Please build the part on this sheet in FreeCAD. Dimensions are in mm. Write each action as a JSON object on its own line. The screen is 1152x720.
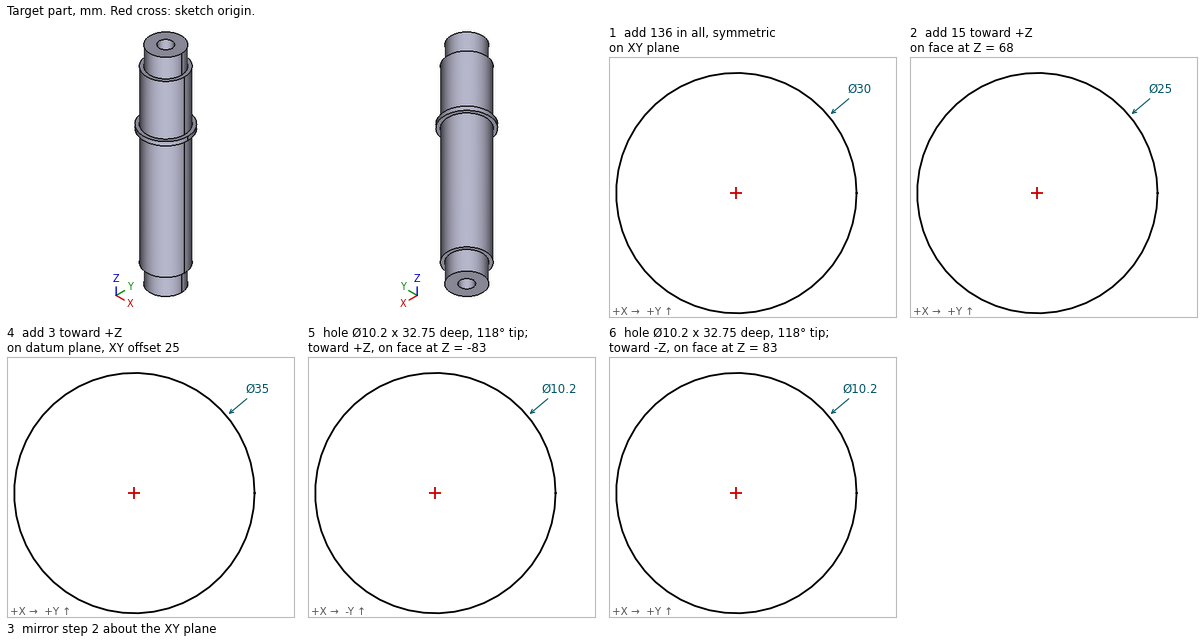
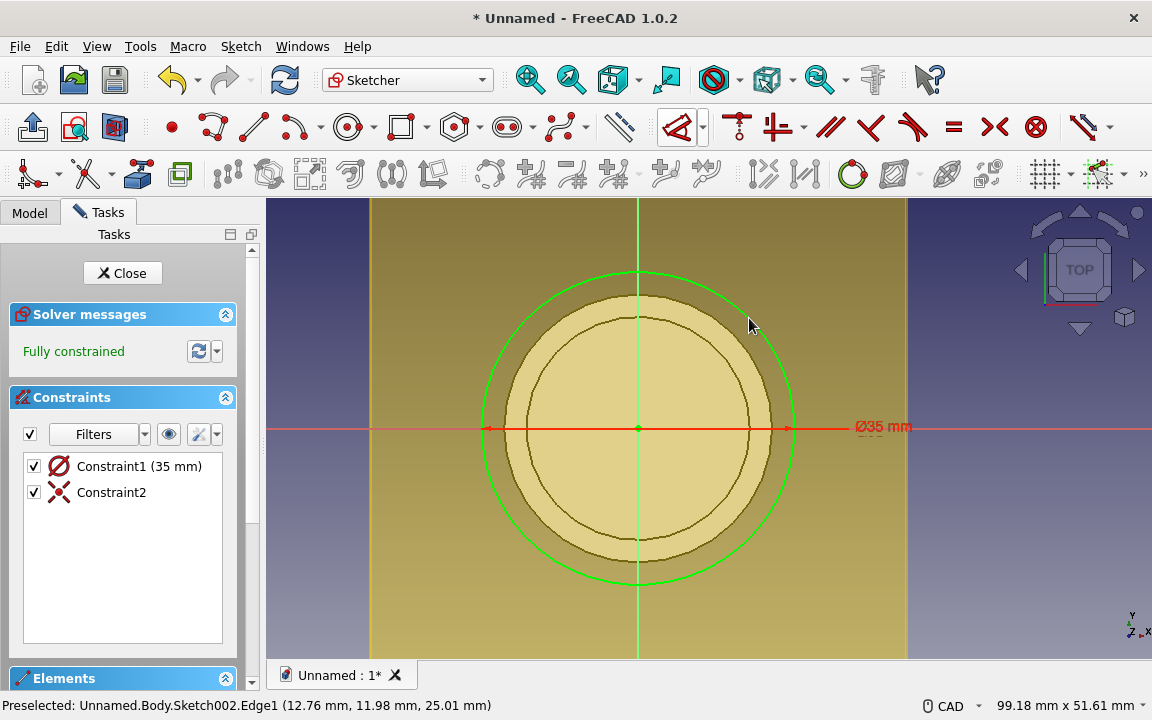
{"action": "left_click", "coordinate": [123, 273]}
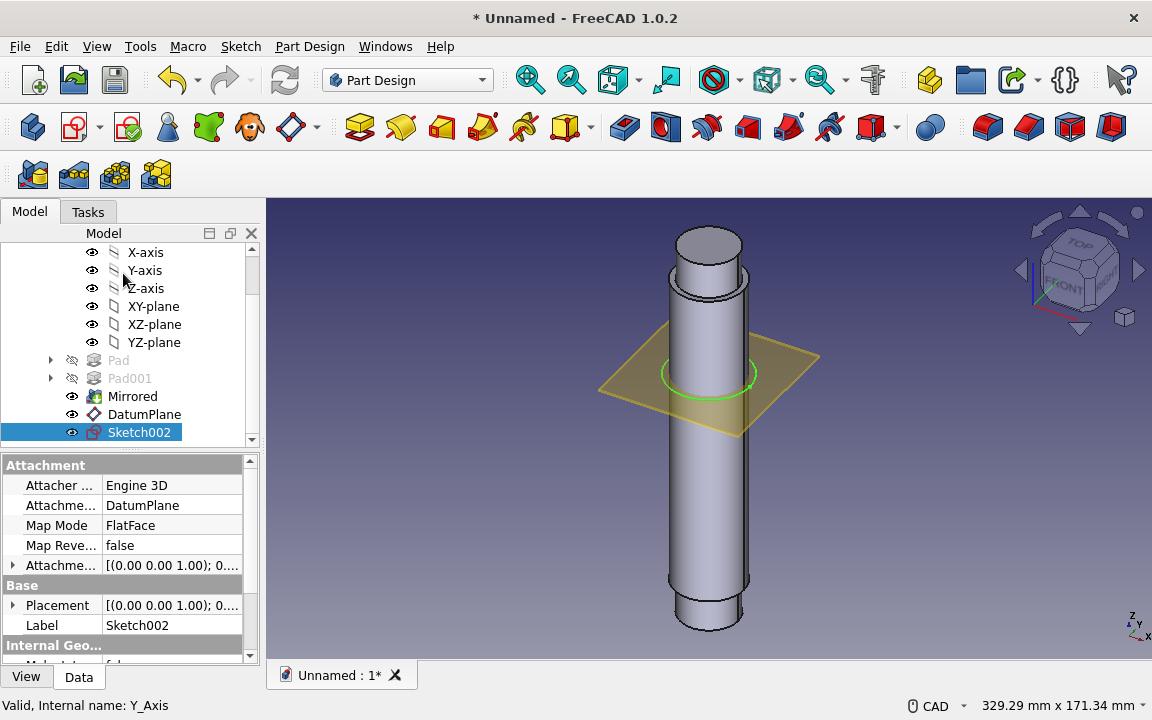
{"action": "left_click", "coordinate": [360, 128]}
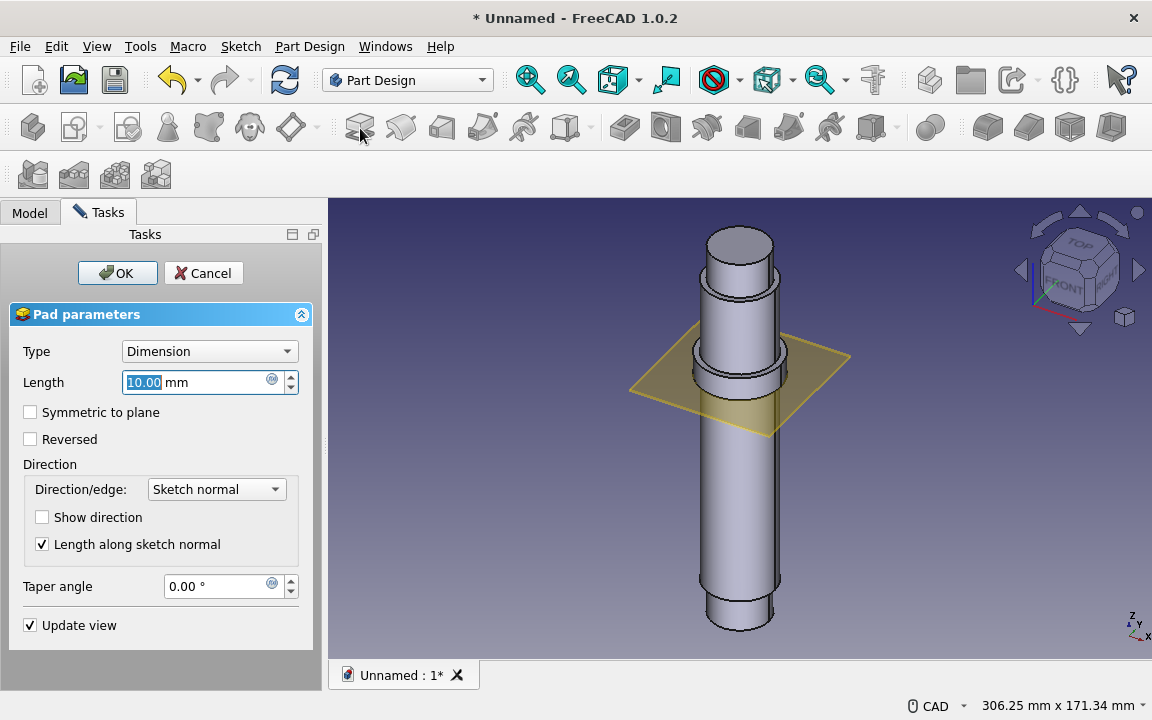
{"action": "type", "text": "3"}
{"action": "key", "text": "Tab"}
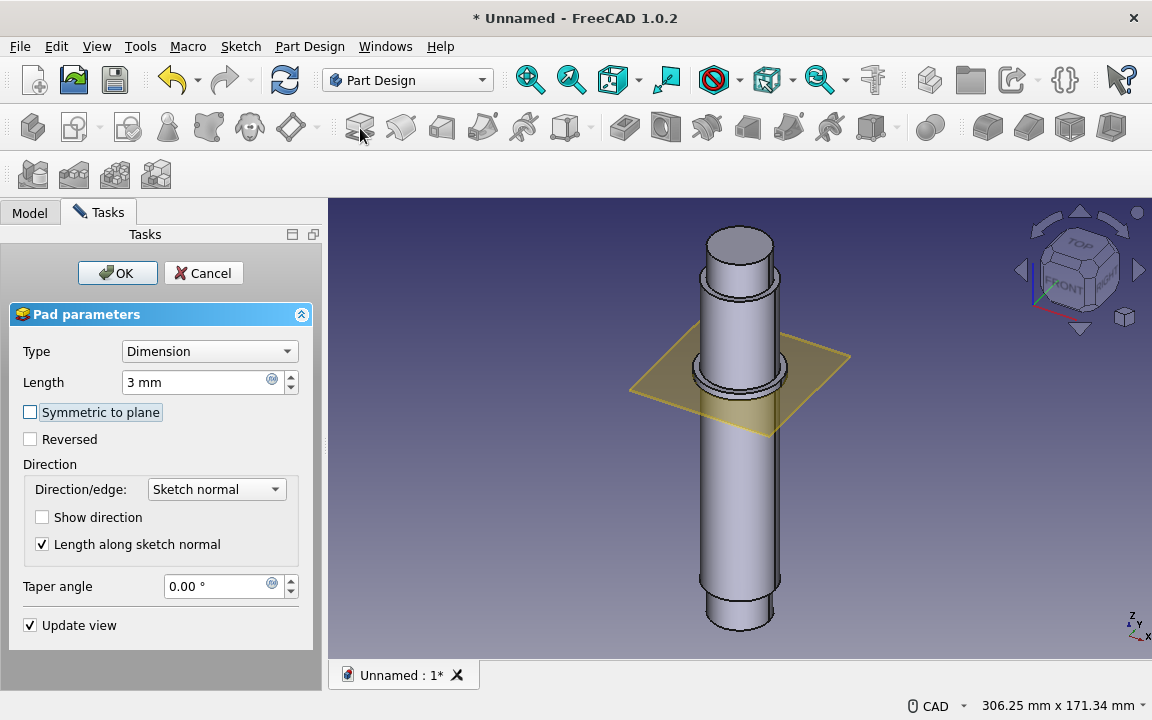
{"action": "left_click", "coordinate": [118, 273]}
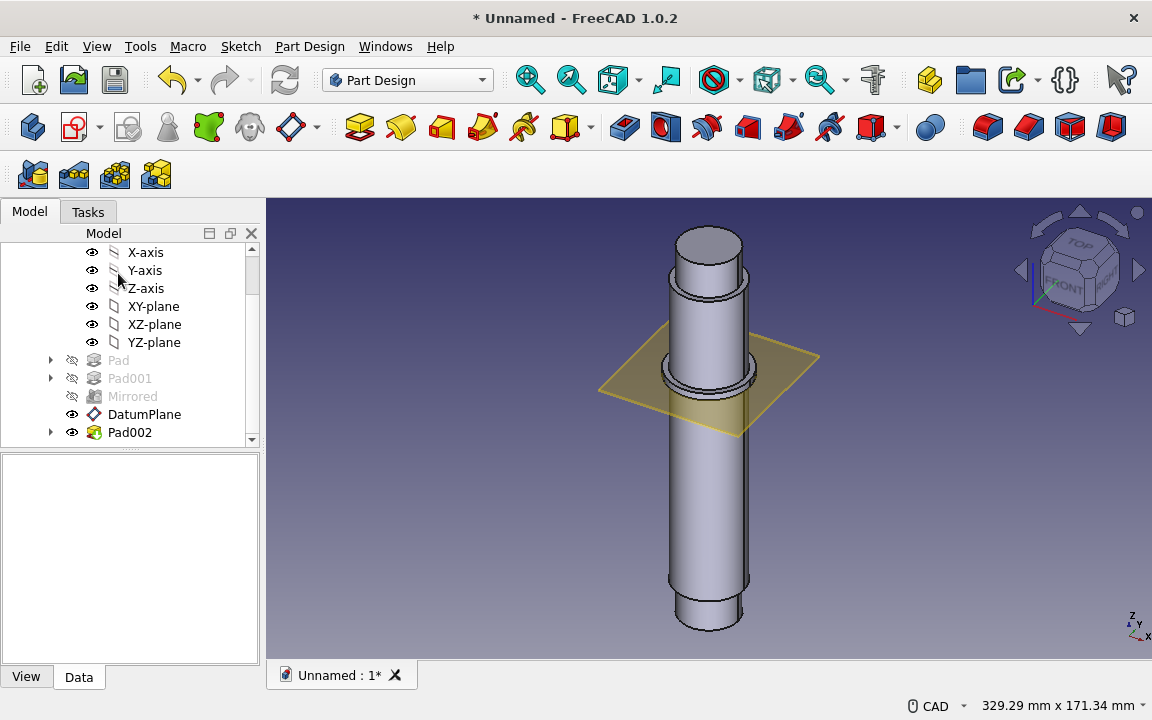
{"action": "left_click", "coordinate": [117, 414]}
{"action": "key", "text": "space"}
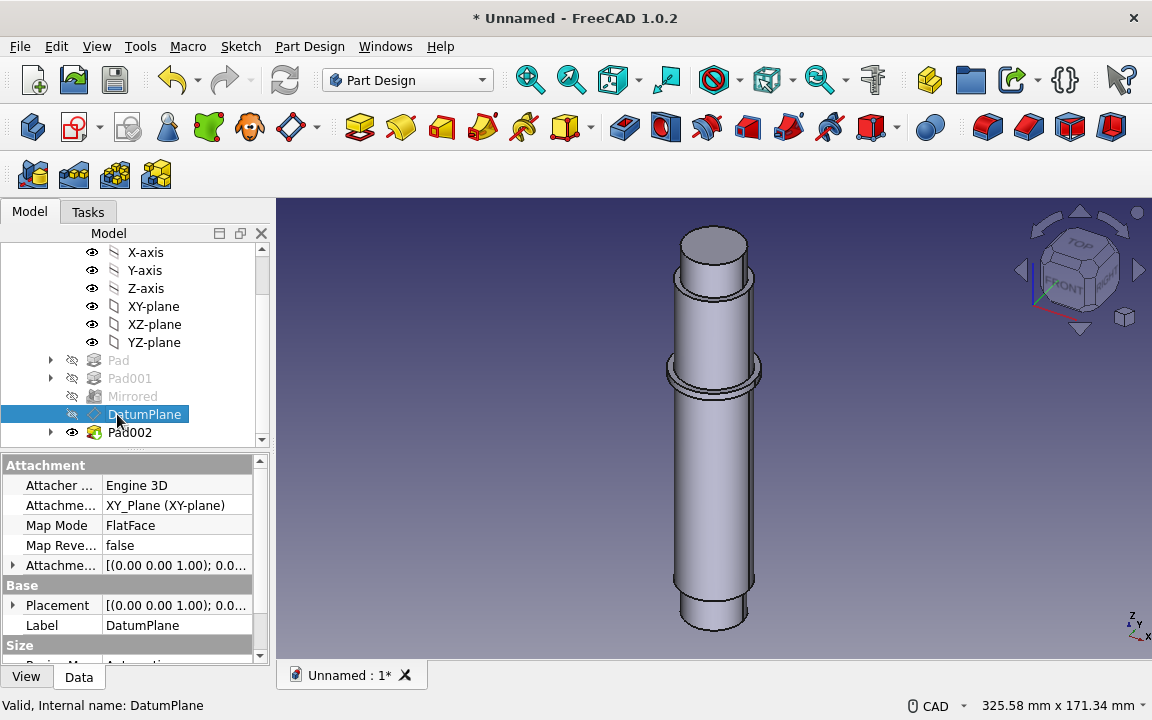
{"action": "key", "text": "5"}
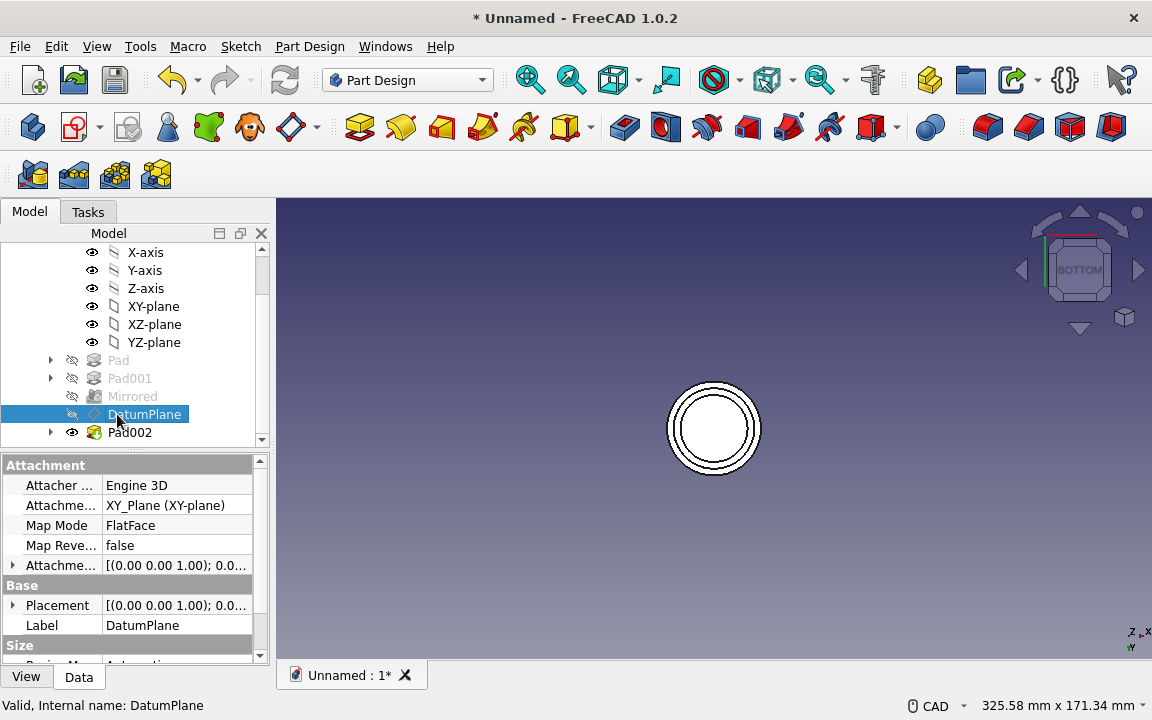
{"action": "left_click", "coordinate": [531, 80]}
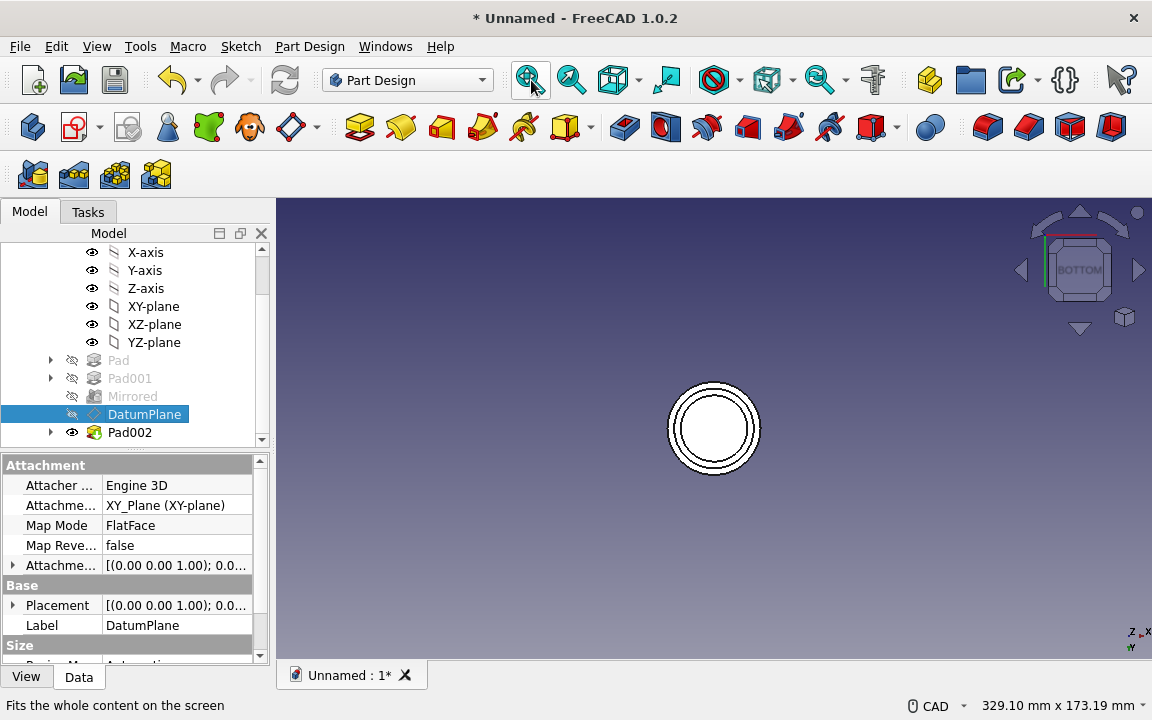
{"action": "left_click", "coordinate": [714, 427]}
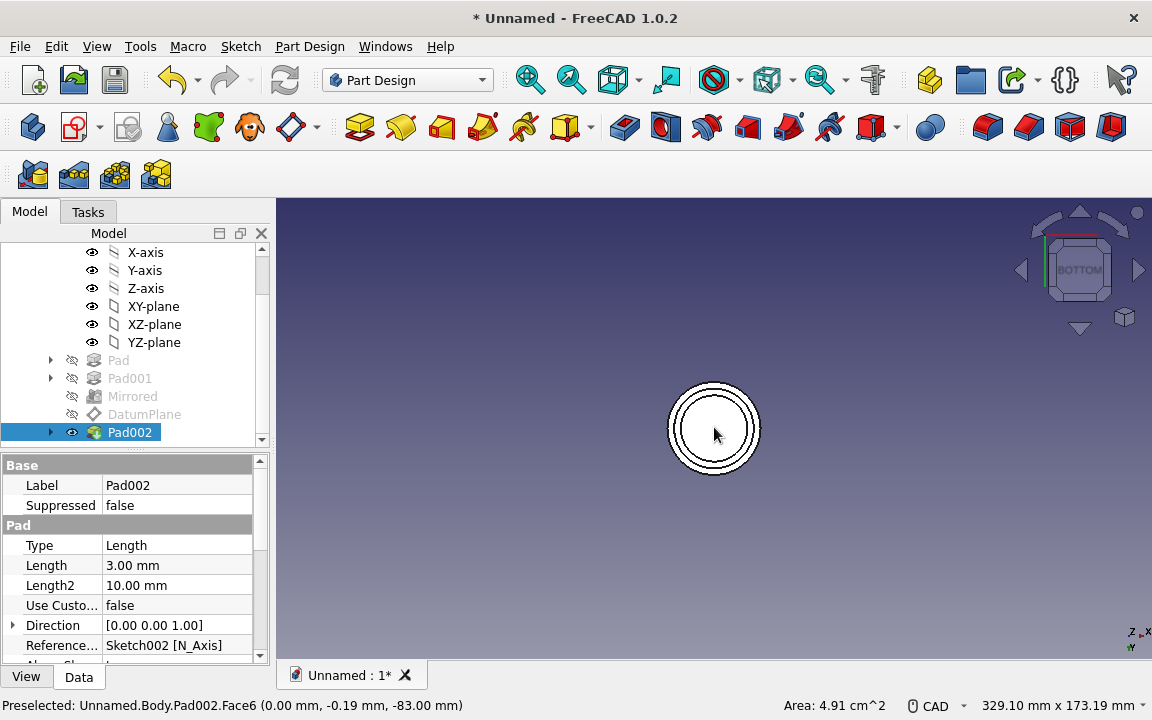
{"action": "left_click", "coordinate": [74, 128]}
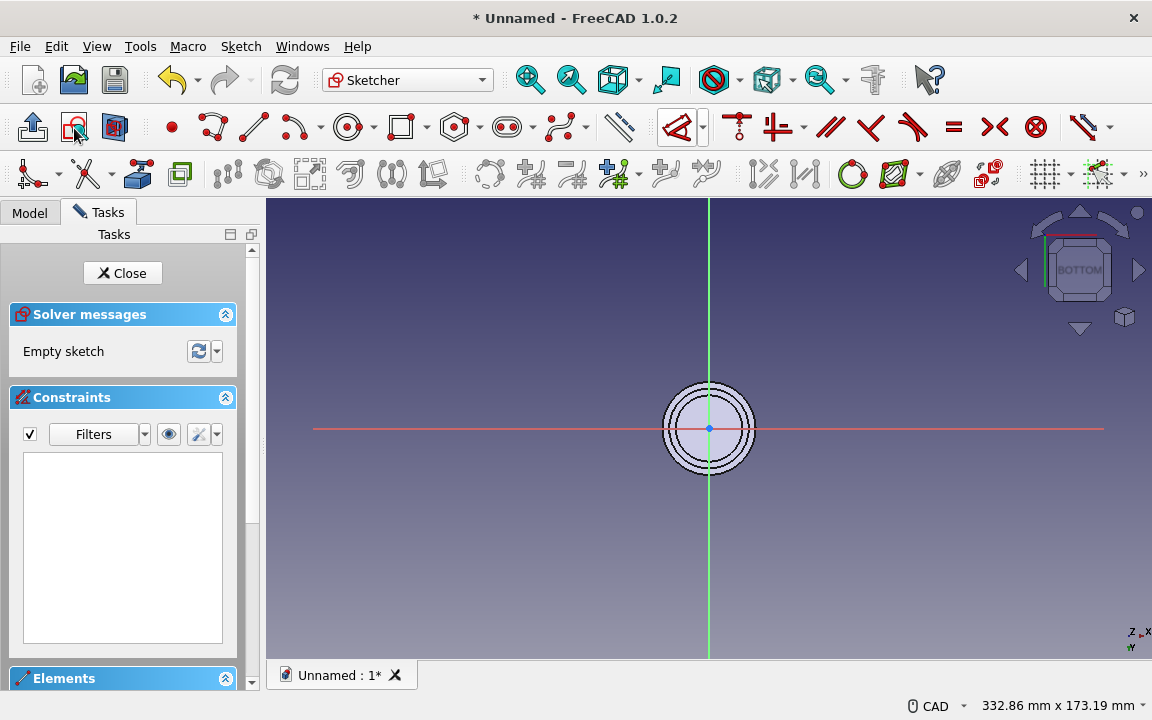
{"action": "scroll", "coordinate": [716, 428], "scroll_direction": "up", "scroll_amount": 12}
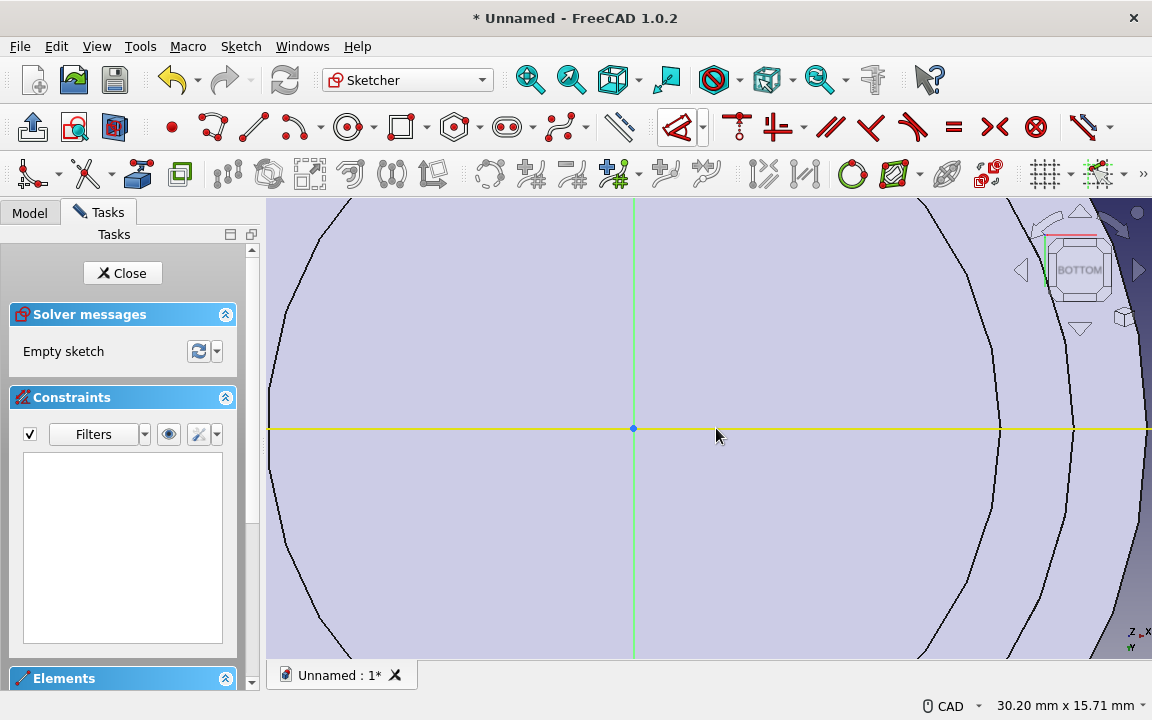
{"action": "left_click", "coordinate": [348, 128]}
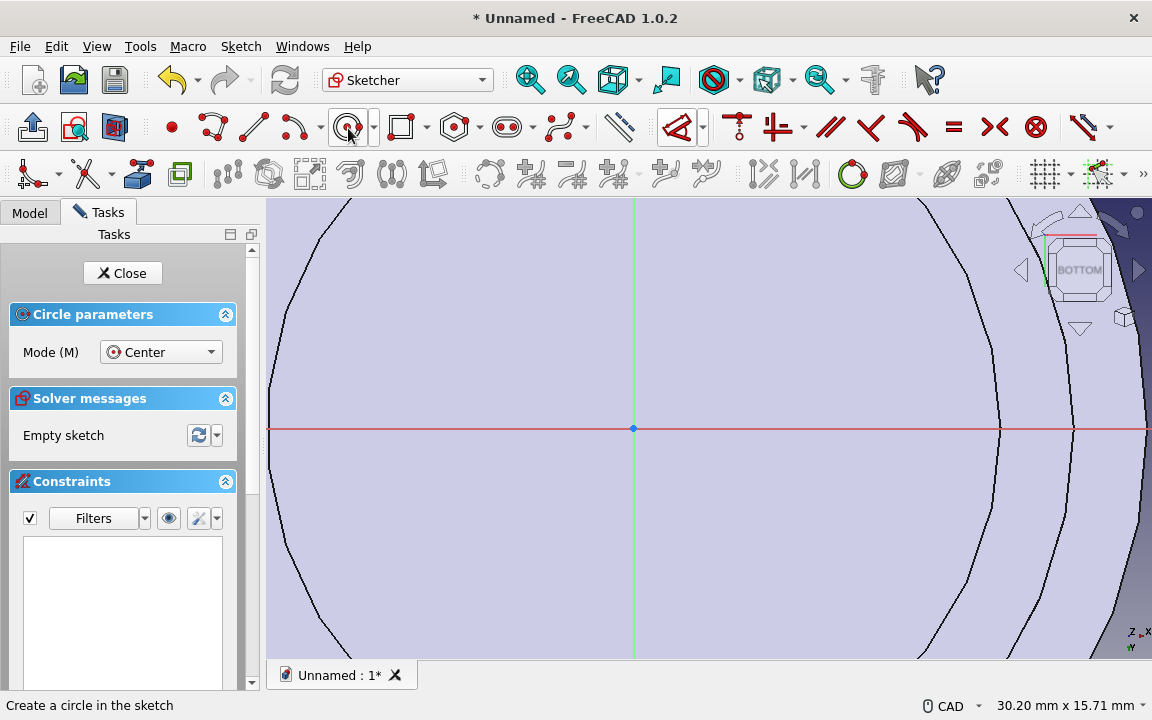
{"action": "left_click", "coordinate": [634, 428]}
{"action": "mouse_move", "coordinate": [740, 323]}